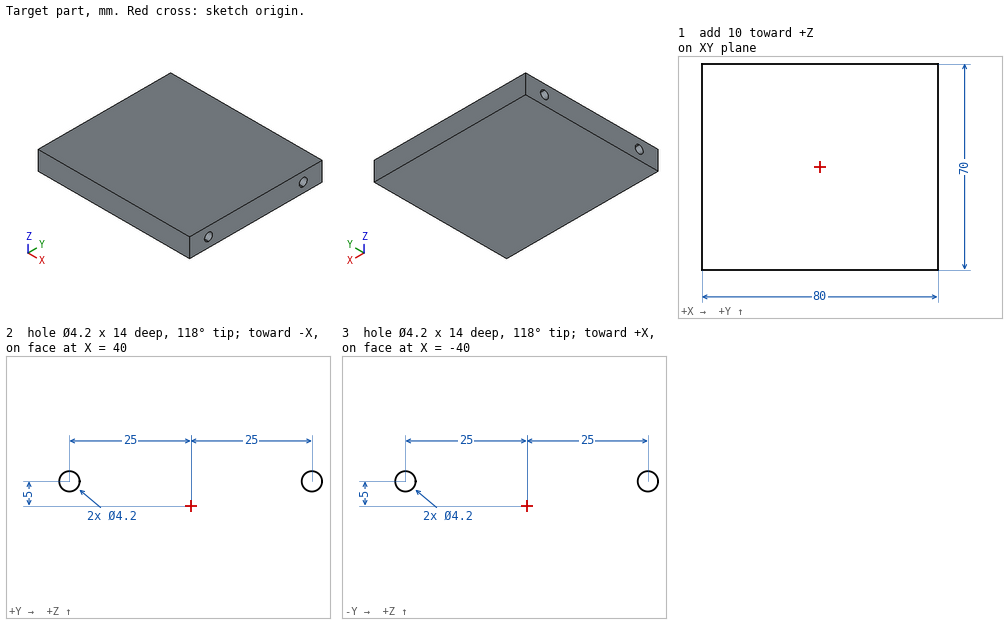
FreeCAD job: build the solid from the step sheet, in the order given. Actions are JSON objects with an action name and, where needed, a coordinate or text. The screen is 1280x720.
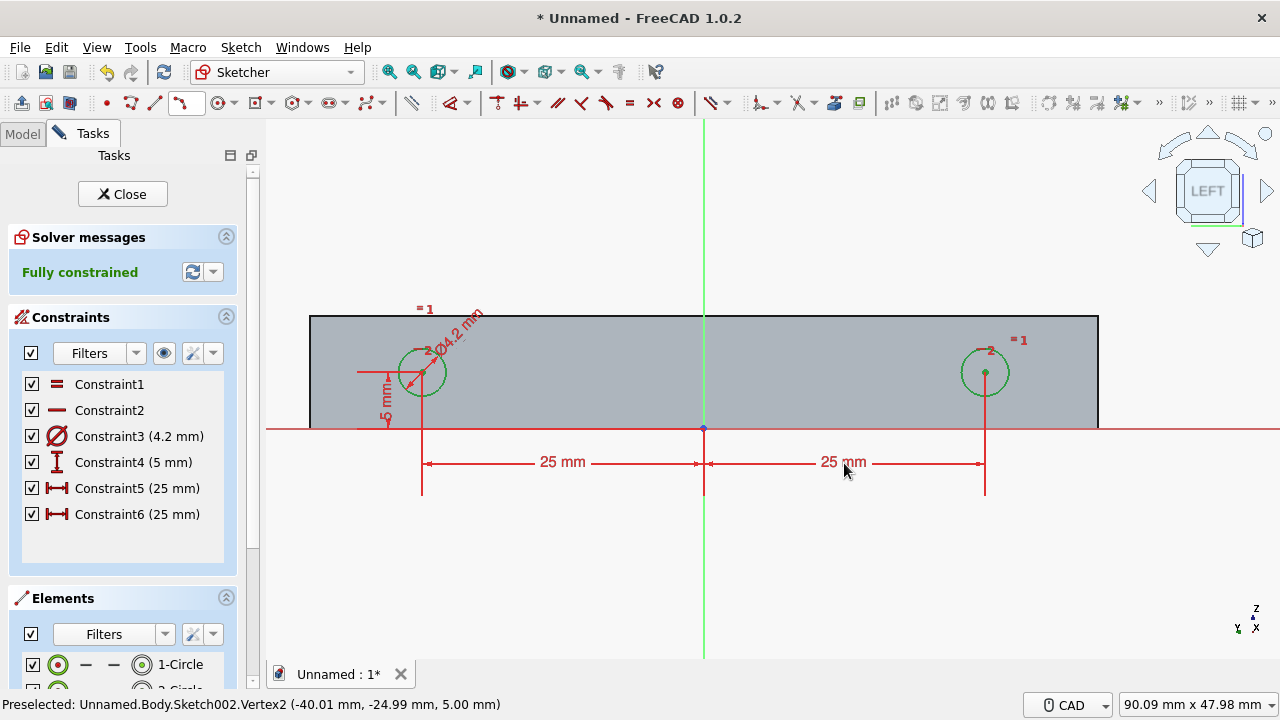
{"action": "left_click", "coordinate": [123, 194]}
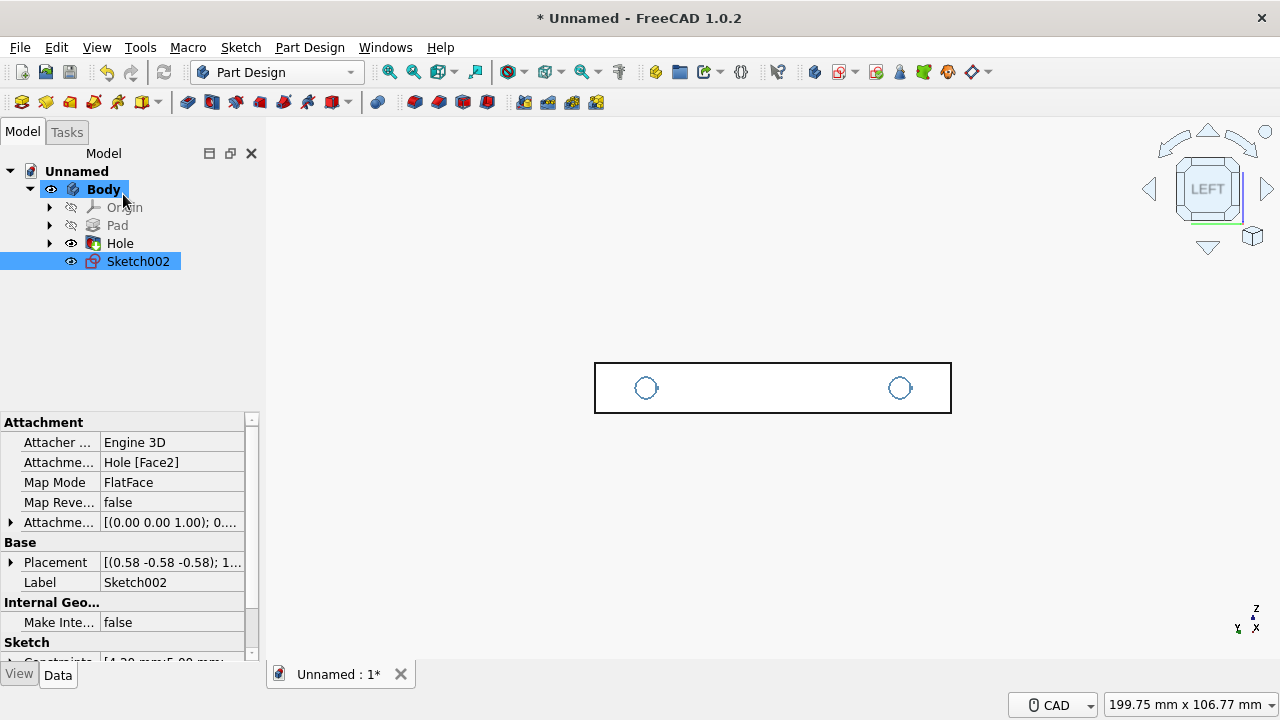
{"action": "left_click", "coordinate": [212, 102]}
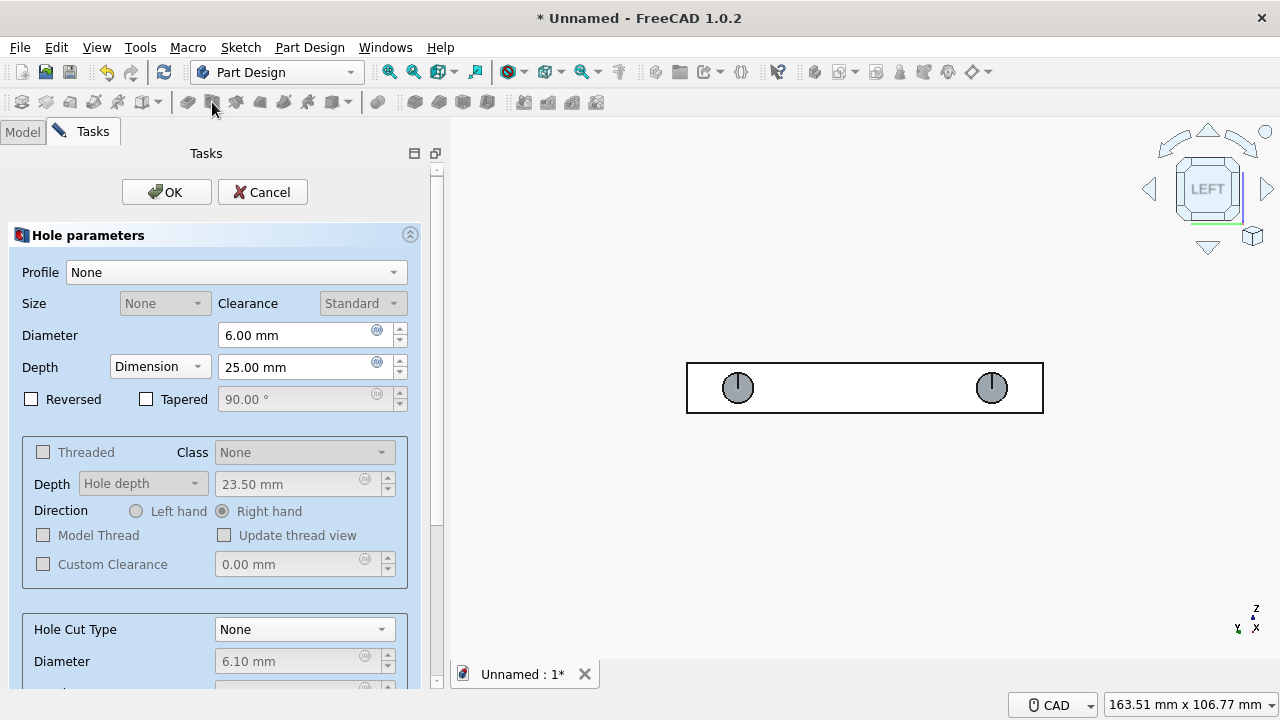
{"action": "triple_click", "coordinate": [305, 335]}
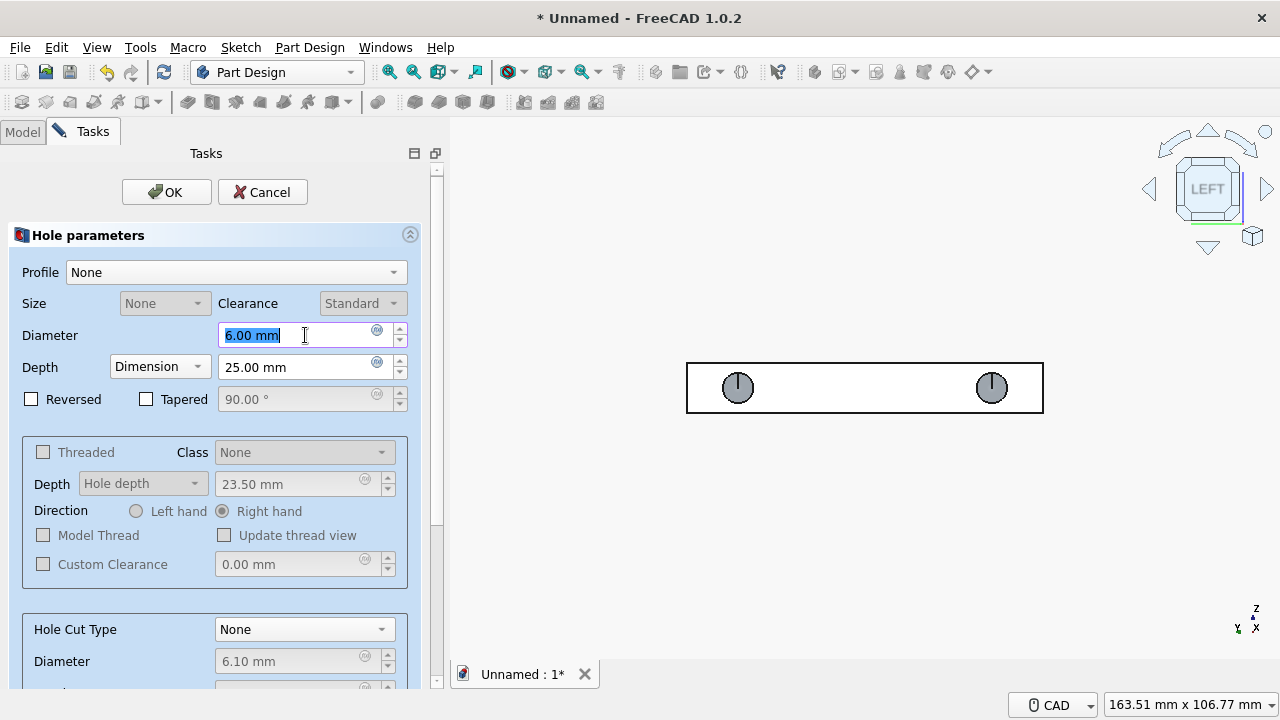
{"action": "type", "text": "4.2"}
{"action": "key", "text": "Tab"}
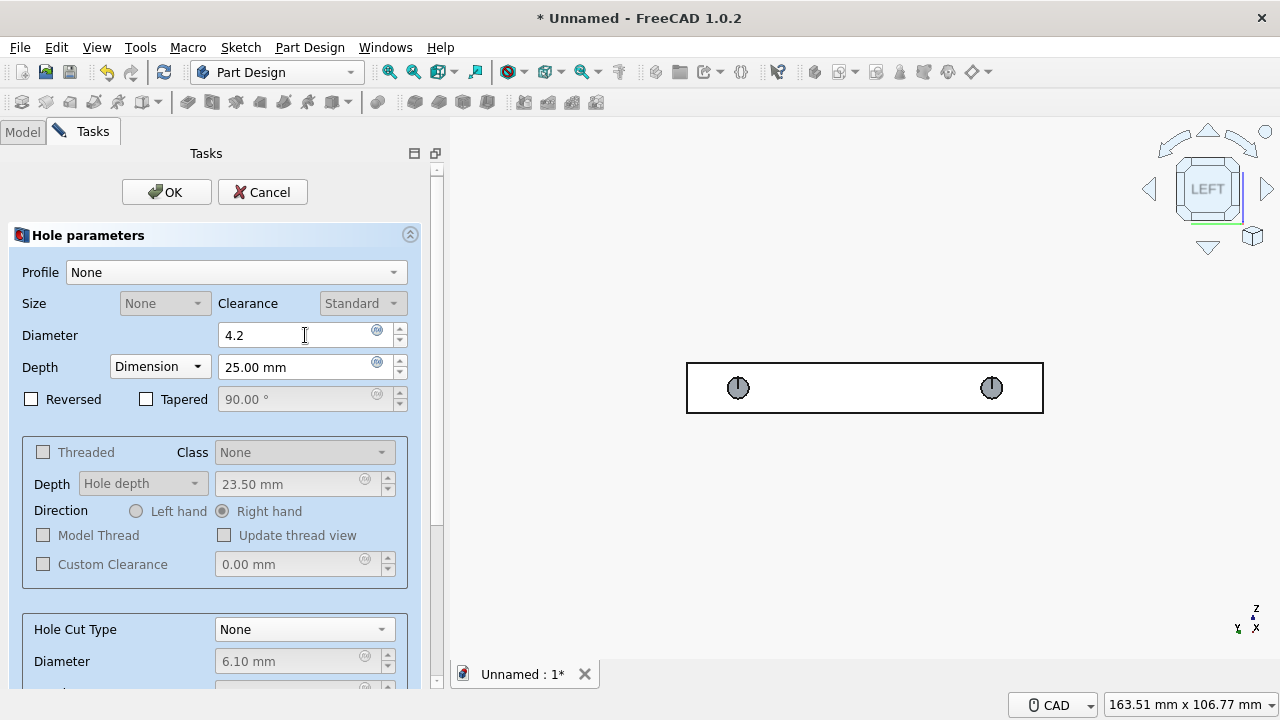
{"action": "triple_click", "coordinate": [305, 367]}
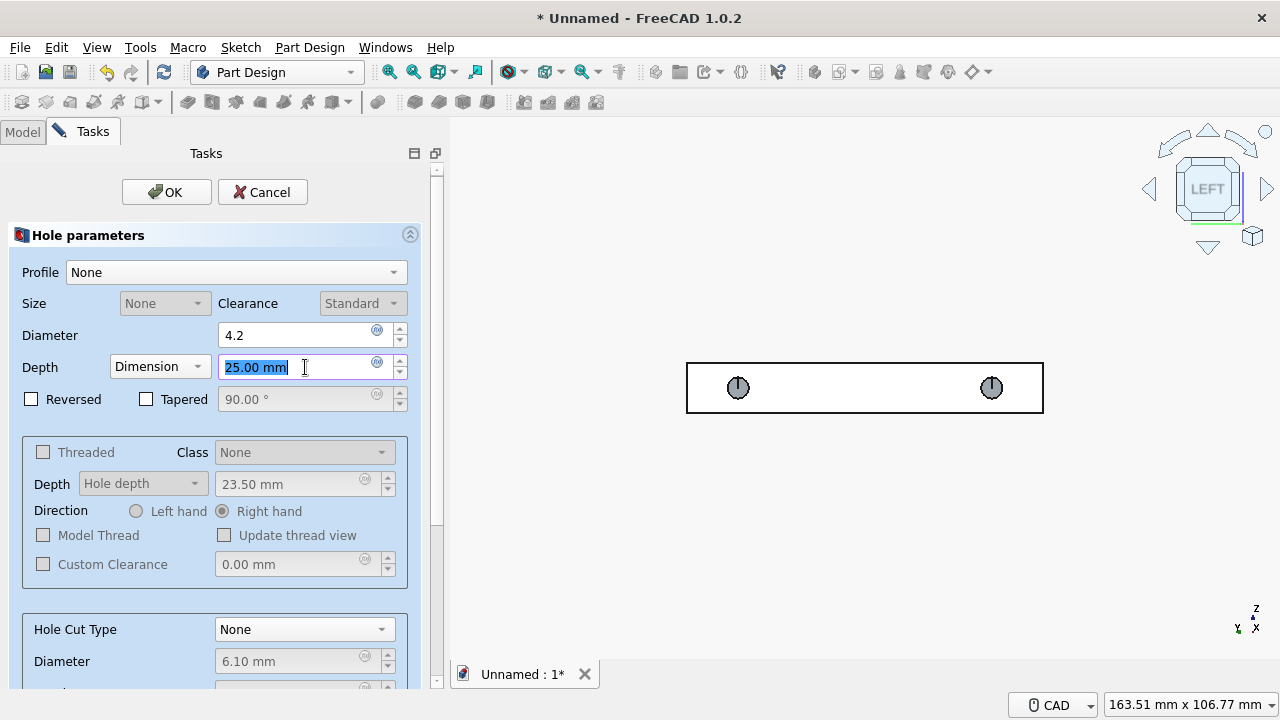
{"action": "type", "text": "14"}
{"action": "key", "text": "Tab"}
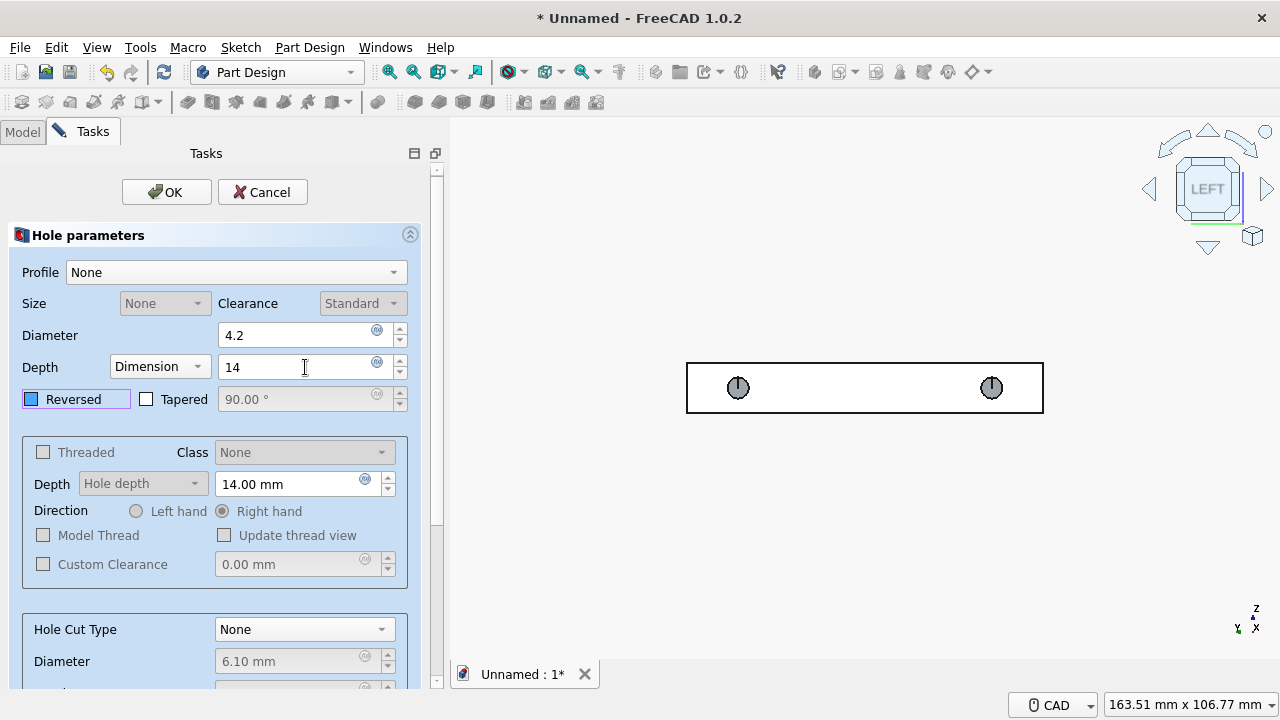
{"action": "left_click", "coordinate": [167, 192]}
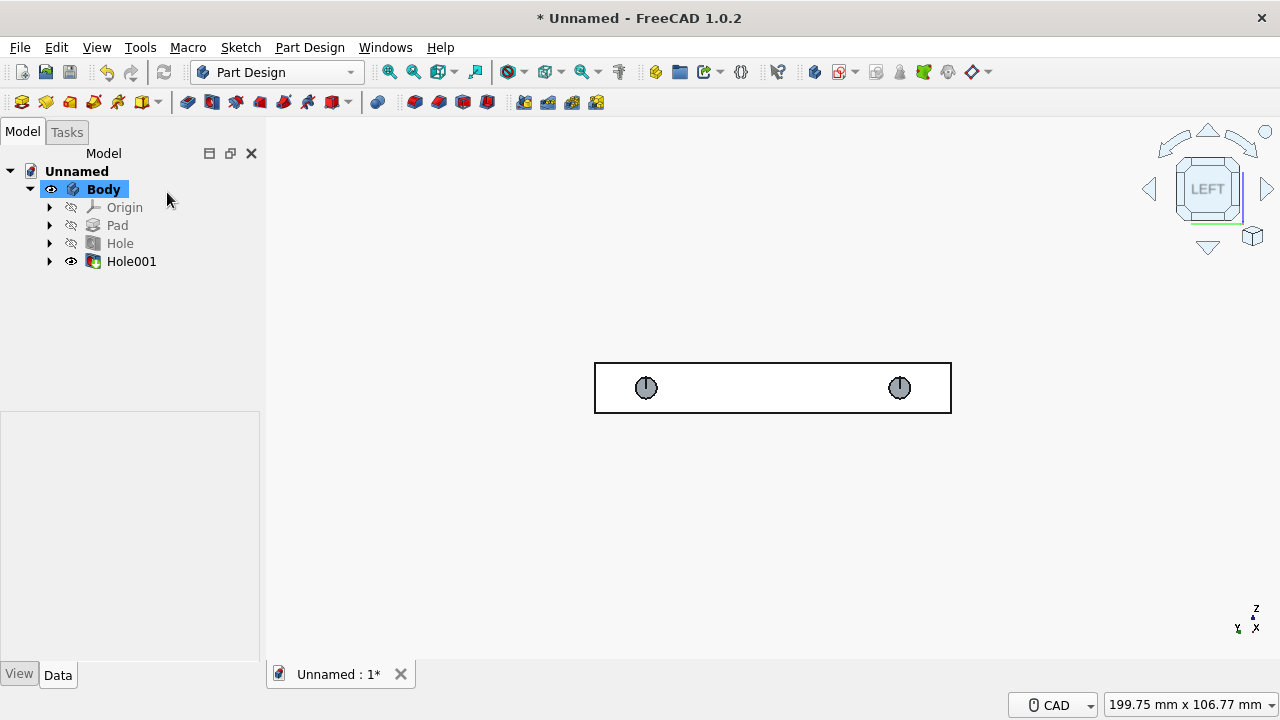
{"action": "key", "text": "0"}